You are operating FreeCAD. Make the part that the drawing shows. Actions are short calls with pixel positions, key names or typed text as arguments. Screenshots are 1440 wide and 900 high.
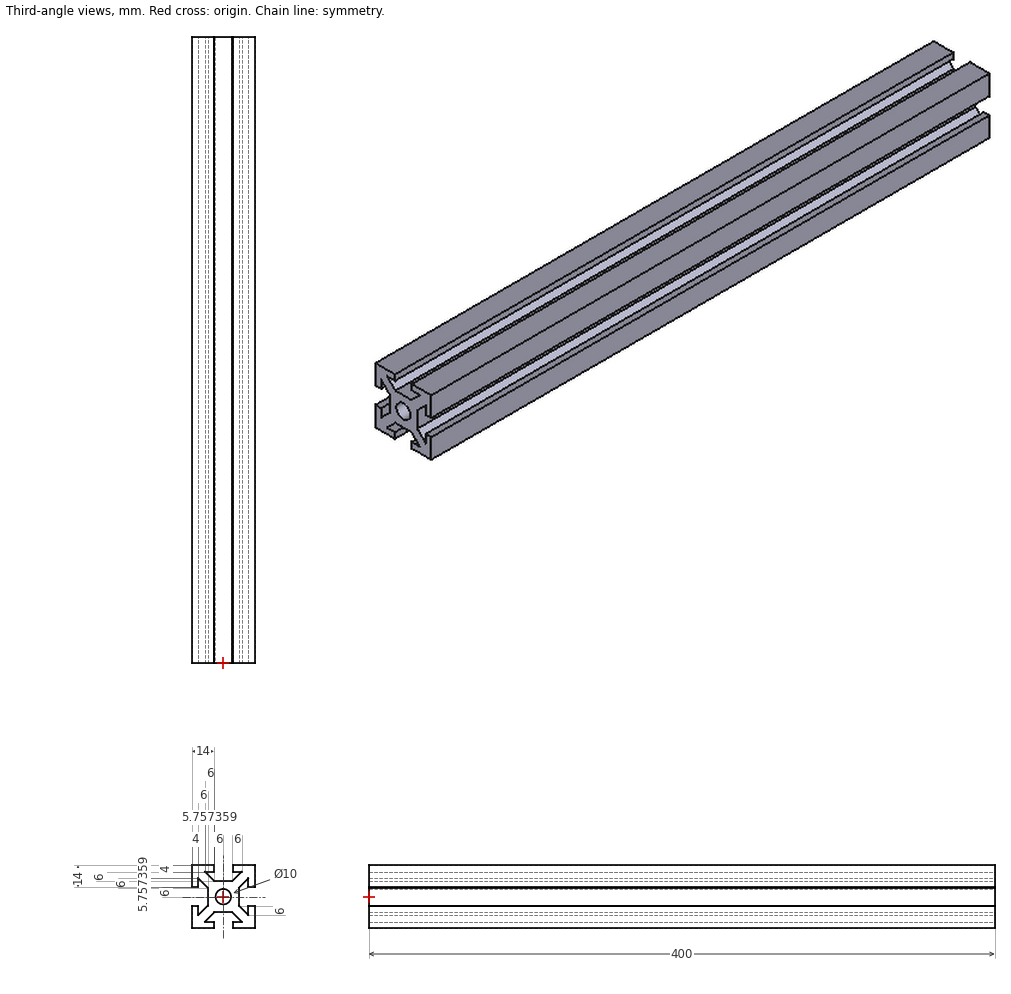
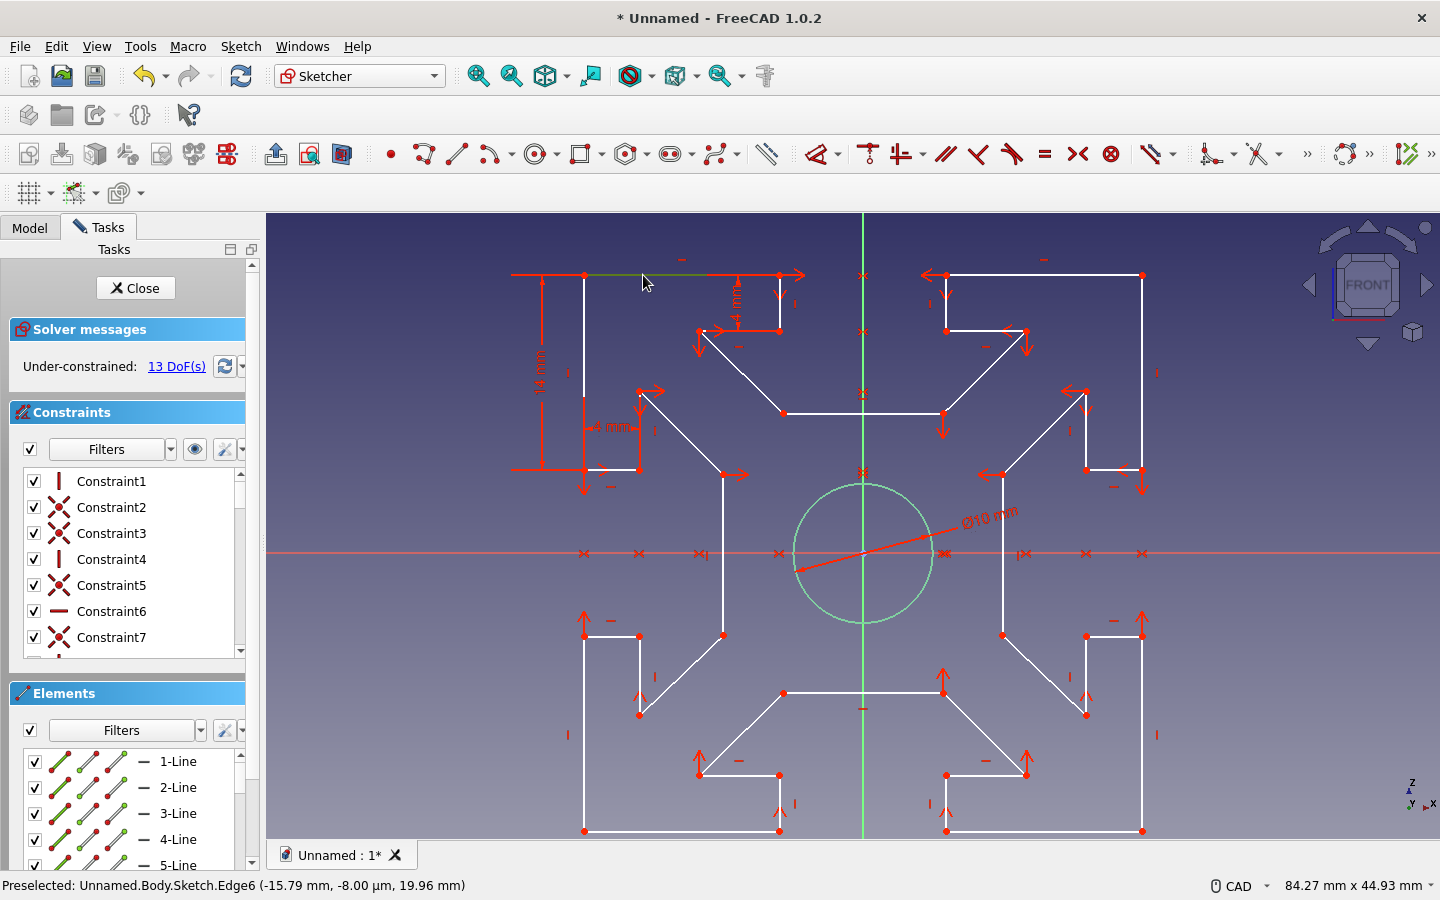
key(l)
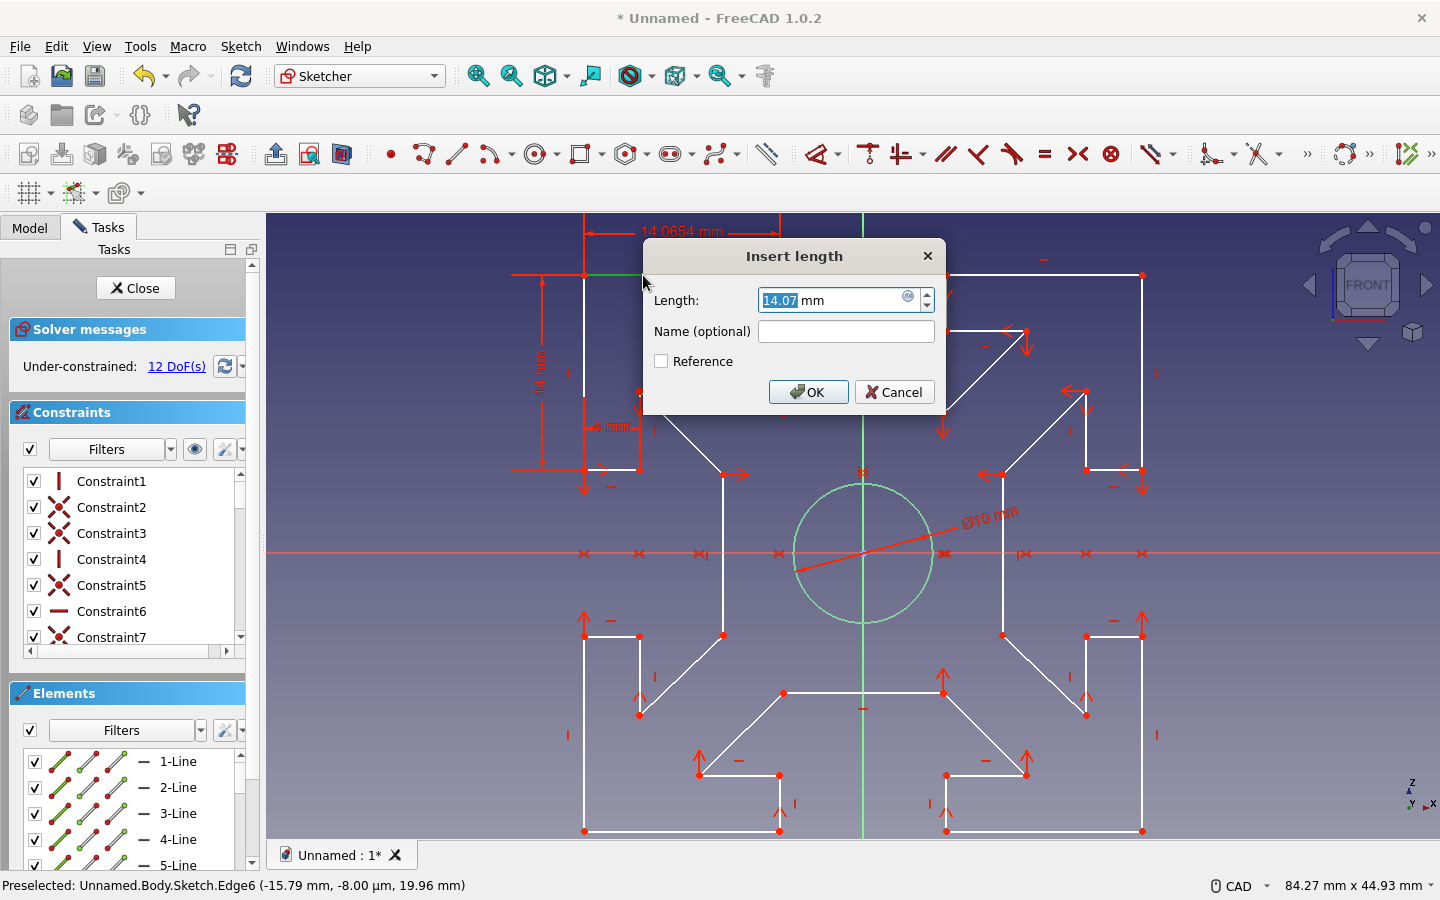
text(14)
key(Return)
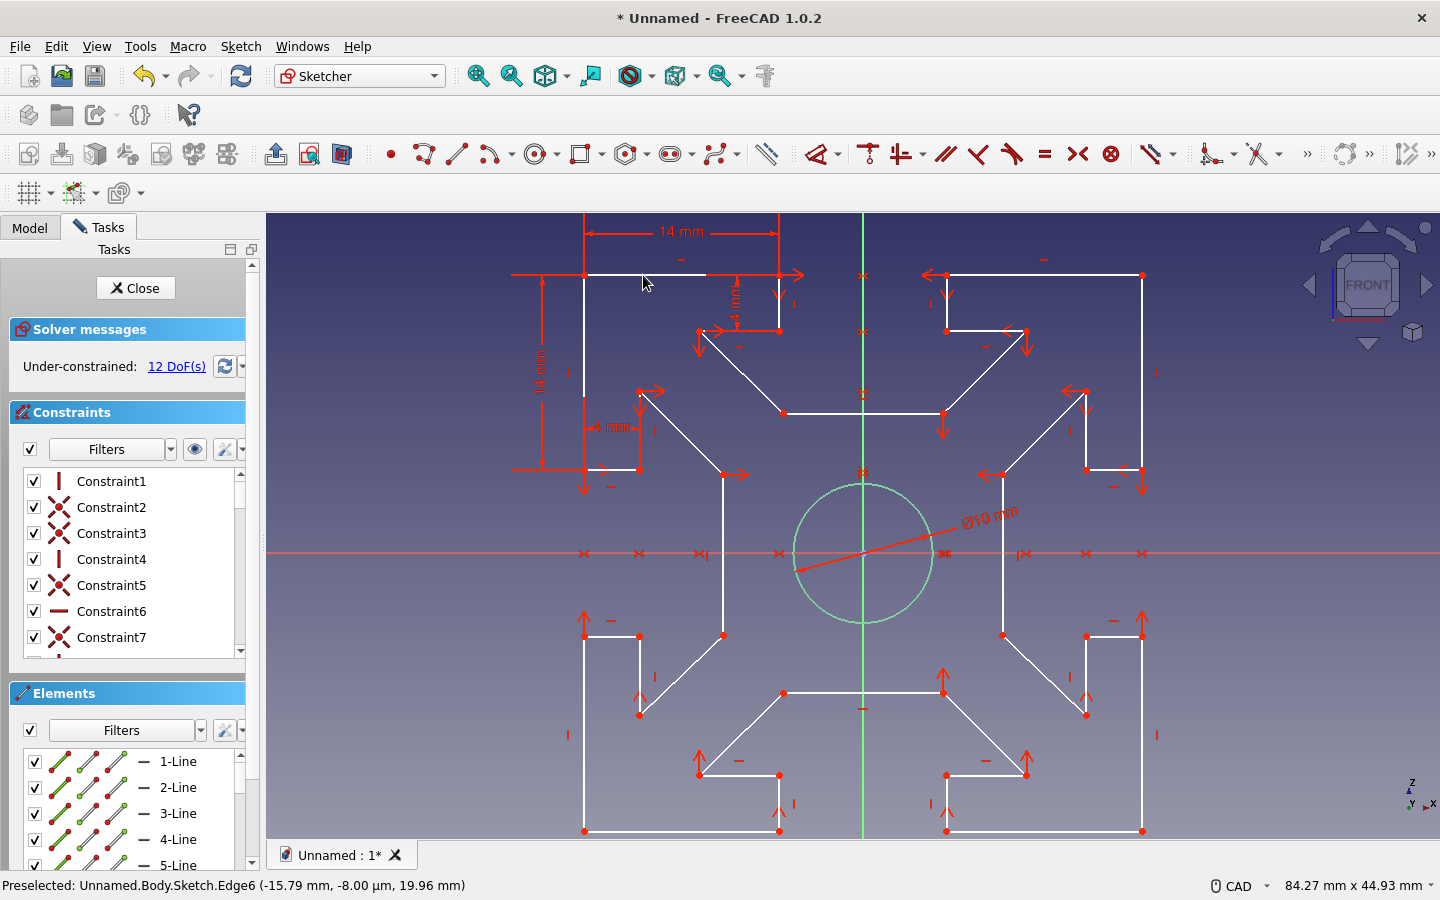
click(640, 470)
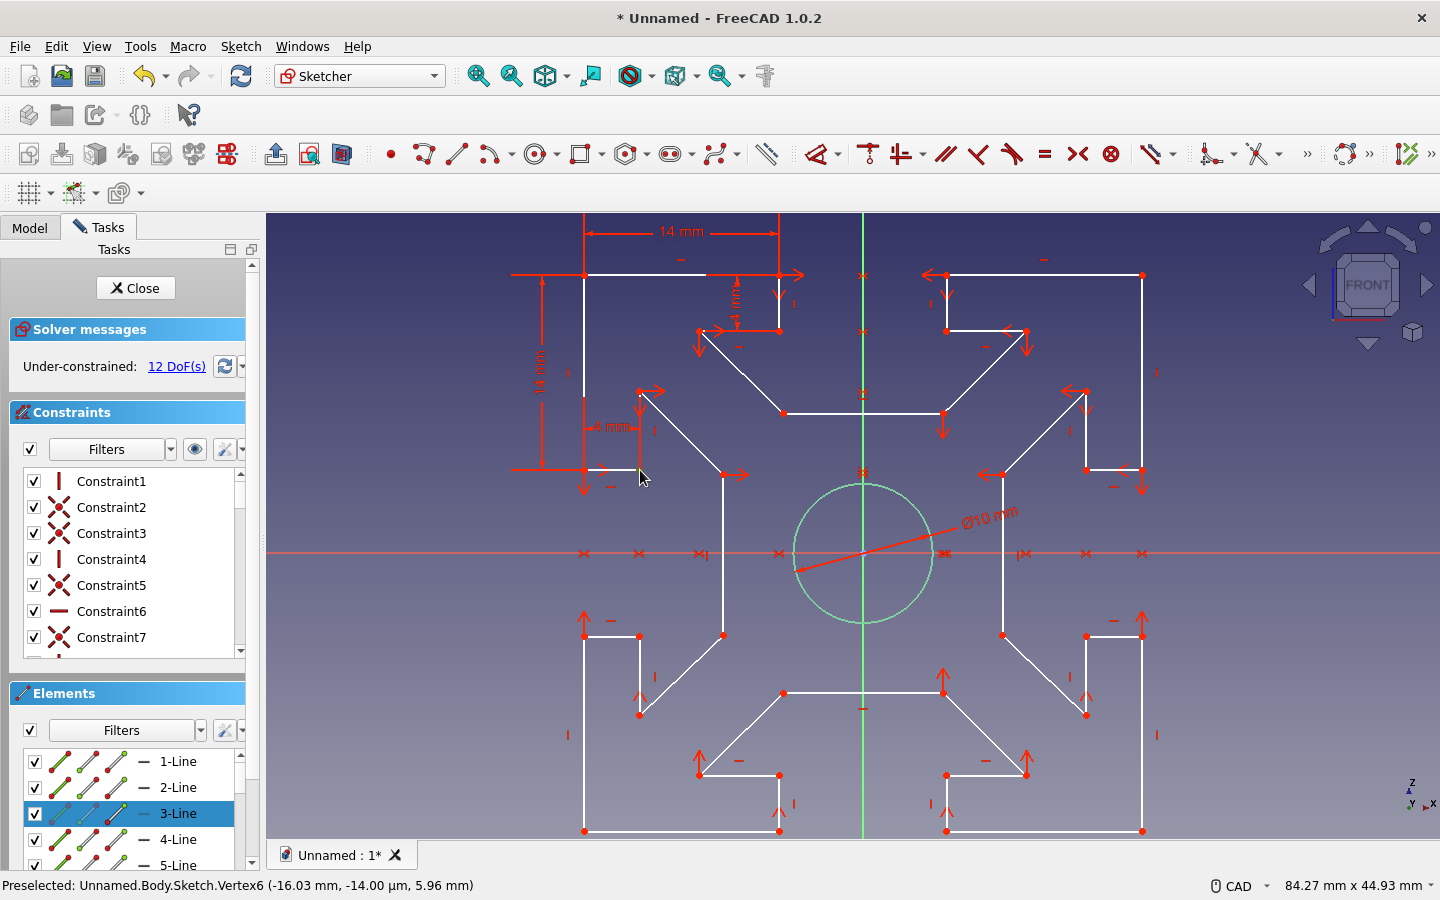
key(i)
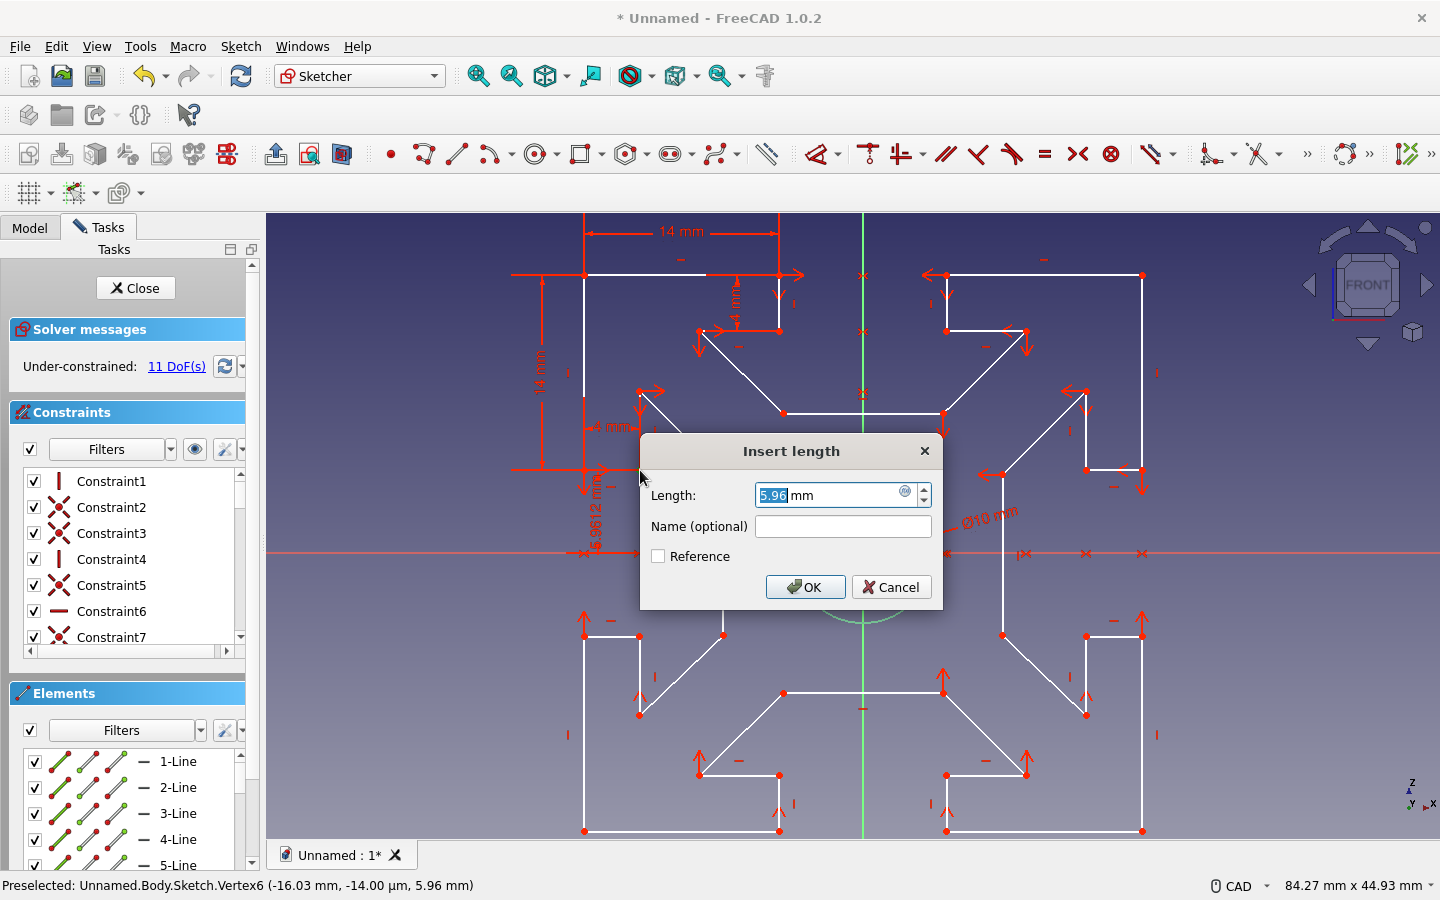
text(6)
key(Return)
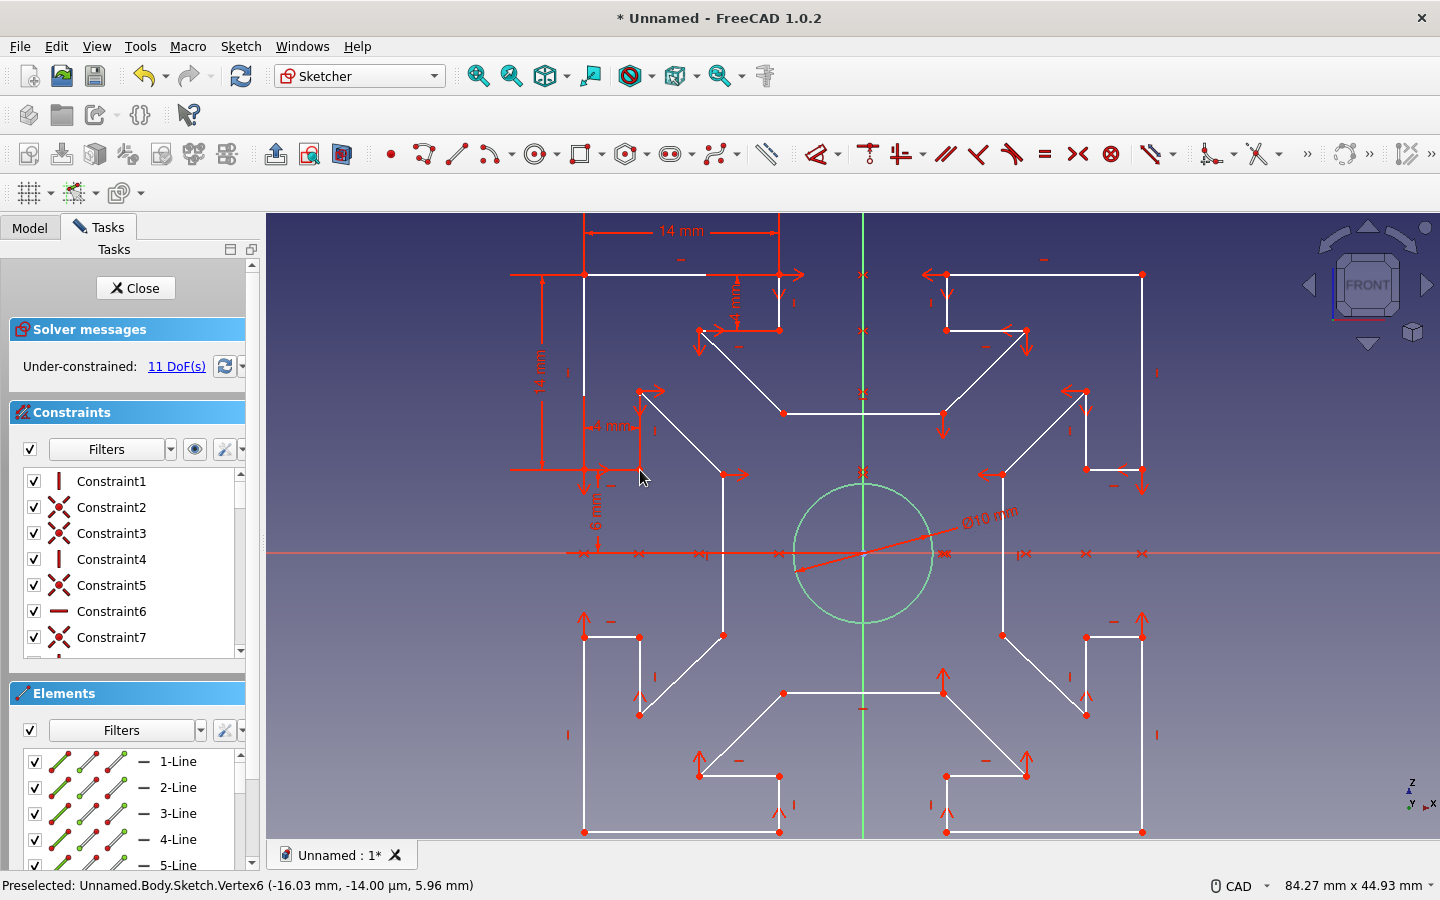
click(779, 275)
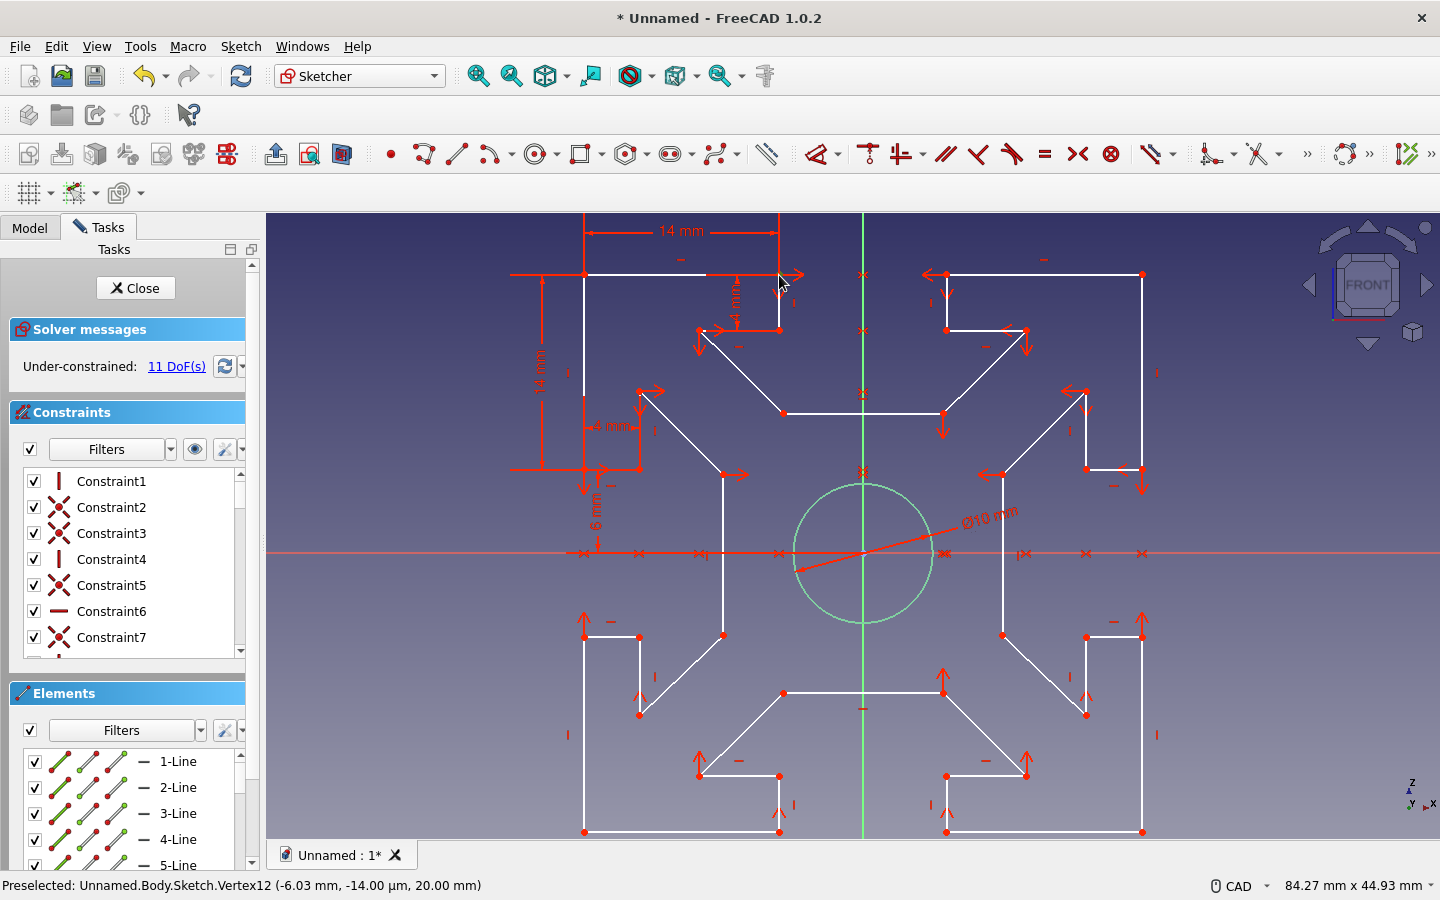
key(l)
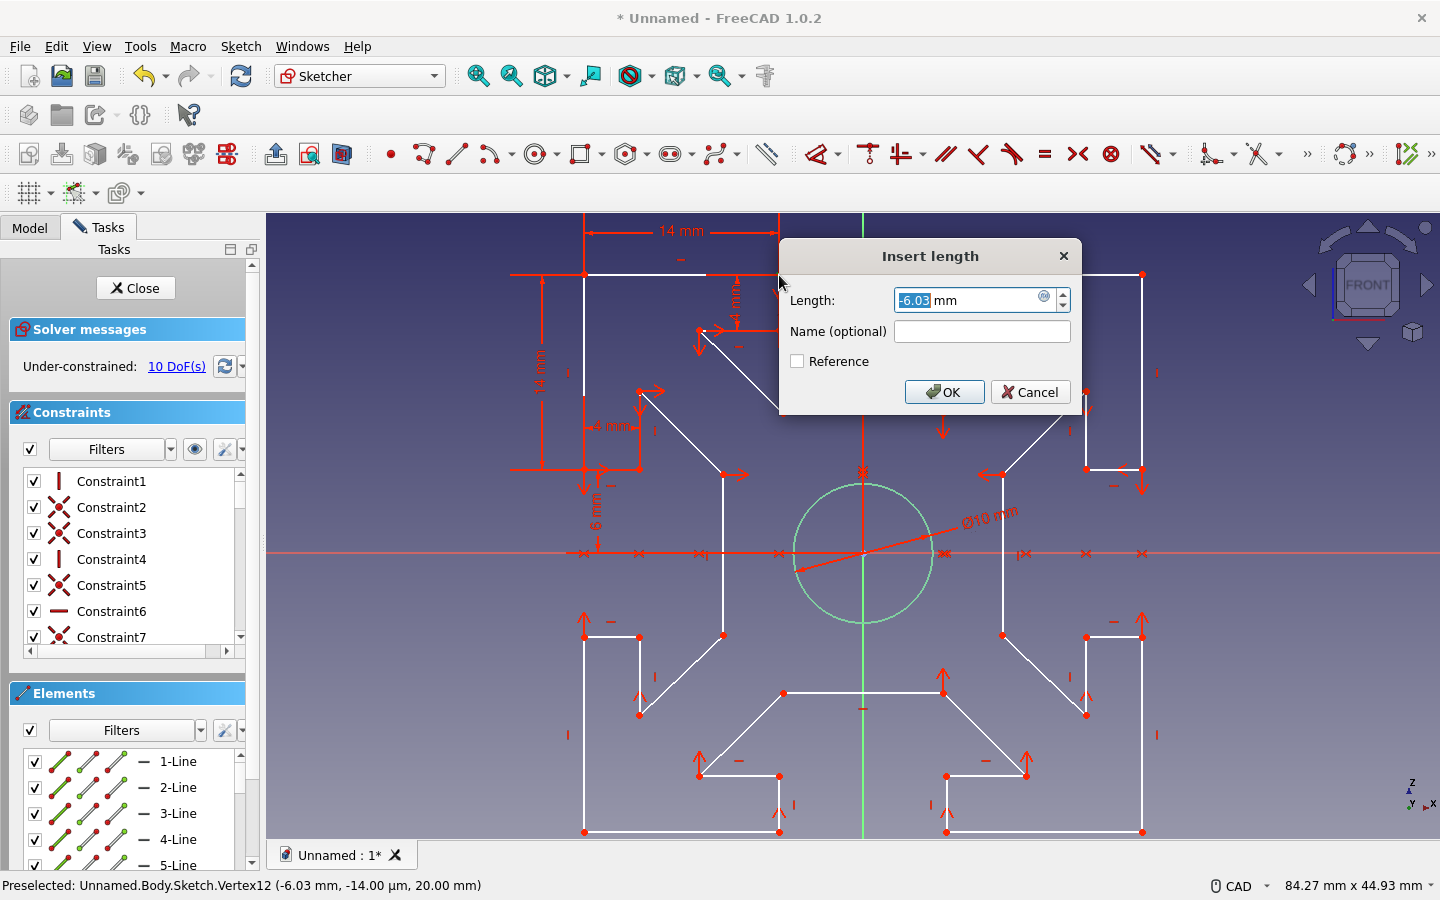
text(-6)
key(Return)